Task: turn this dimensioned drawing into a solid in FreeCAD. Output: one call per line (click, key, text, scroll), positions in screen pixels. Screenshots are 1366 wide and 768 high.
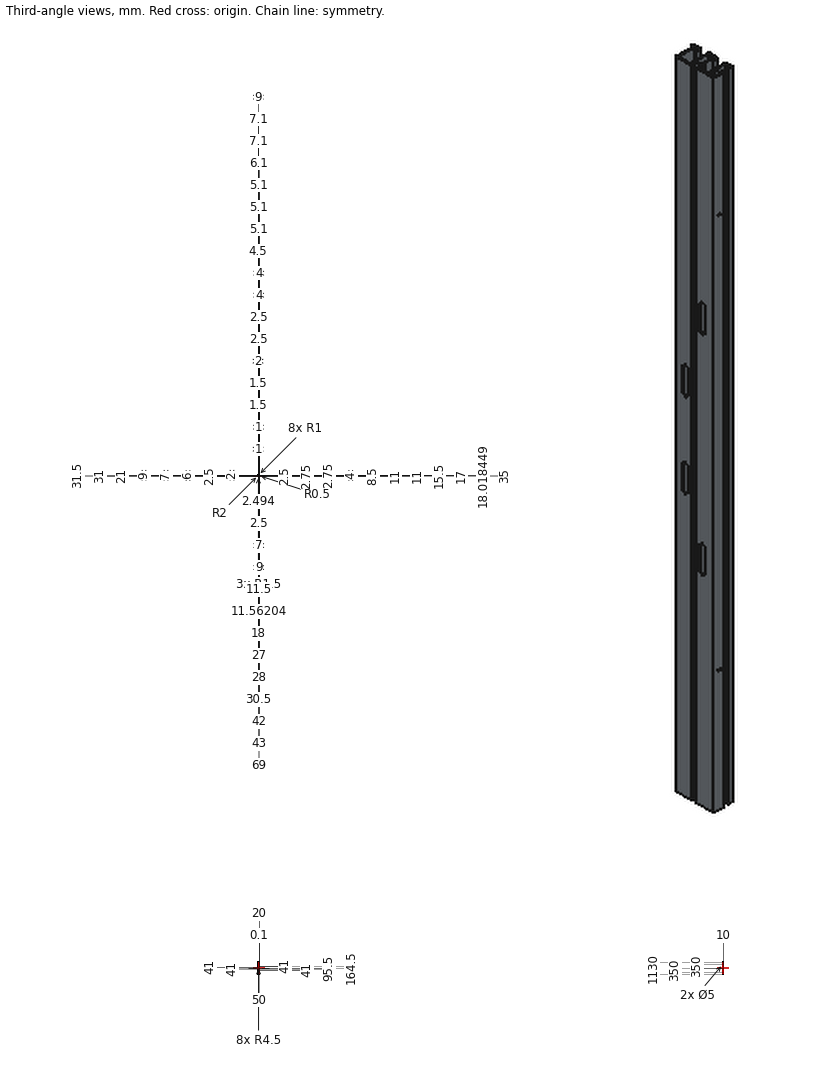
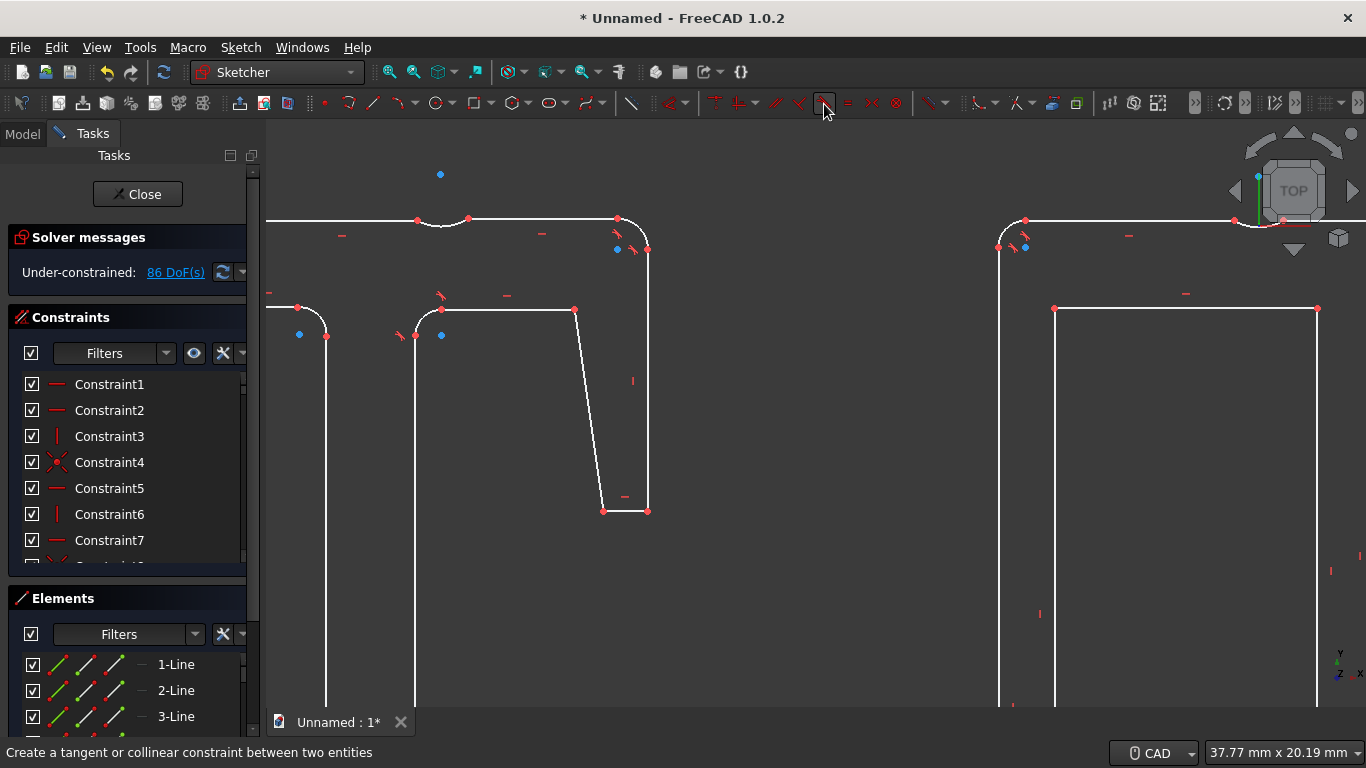
click(373, 221)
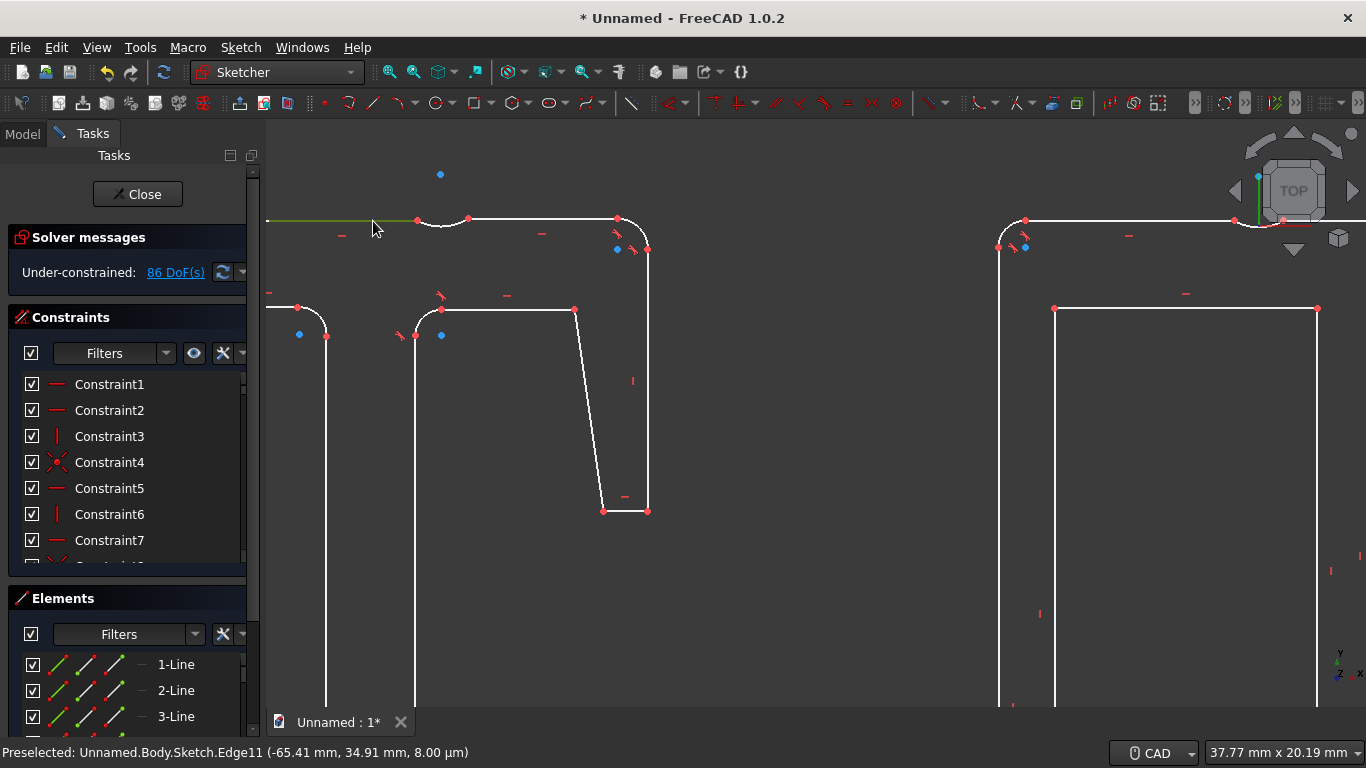
scroll(527, 277, down, 6)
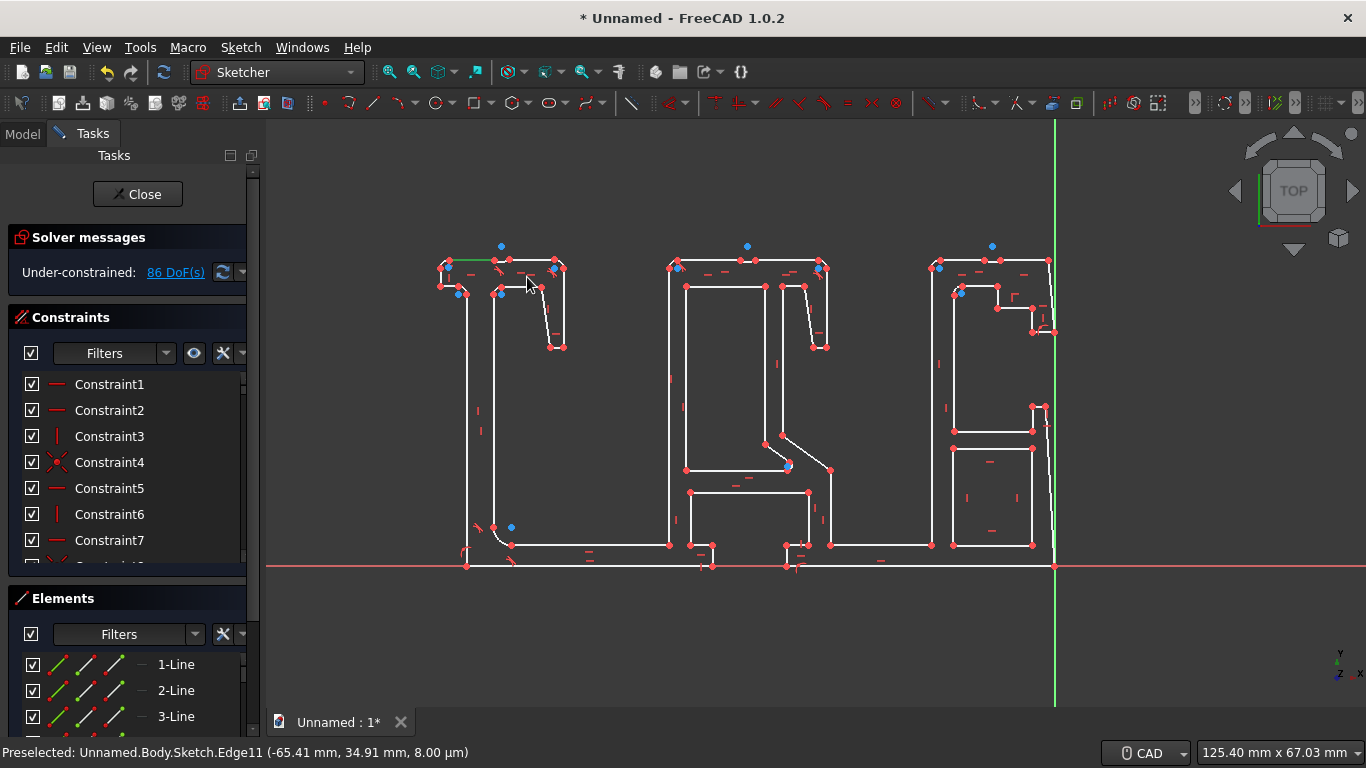
scroll(445, 261, up, 6)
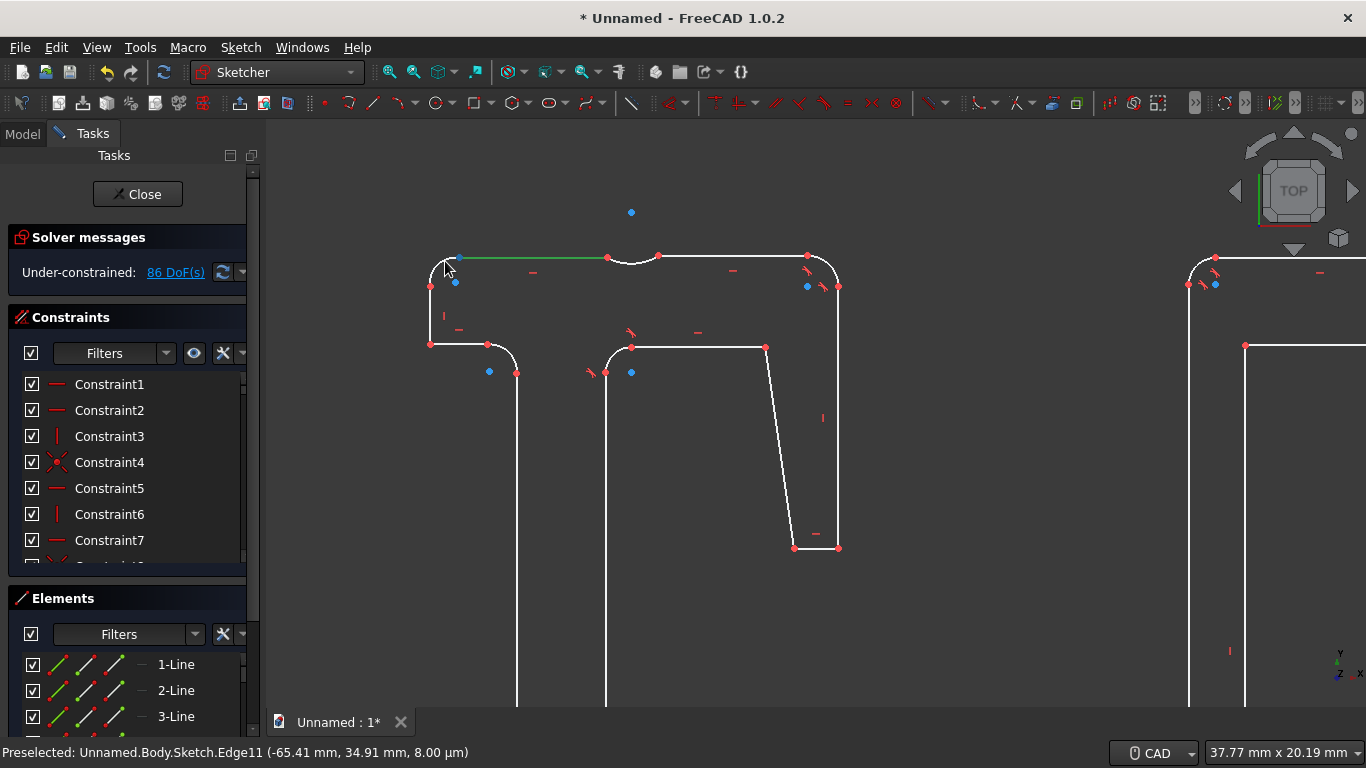
click(445, 260)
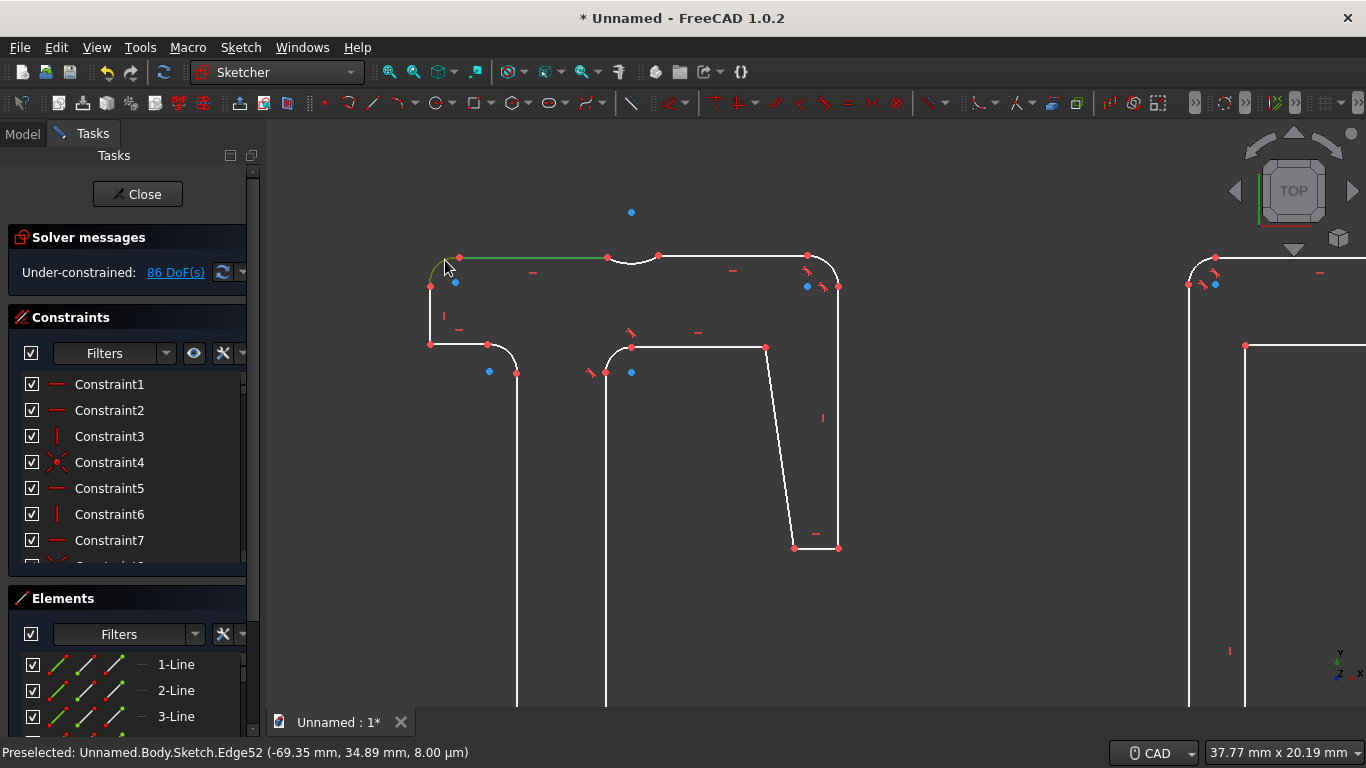
key(t)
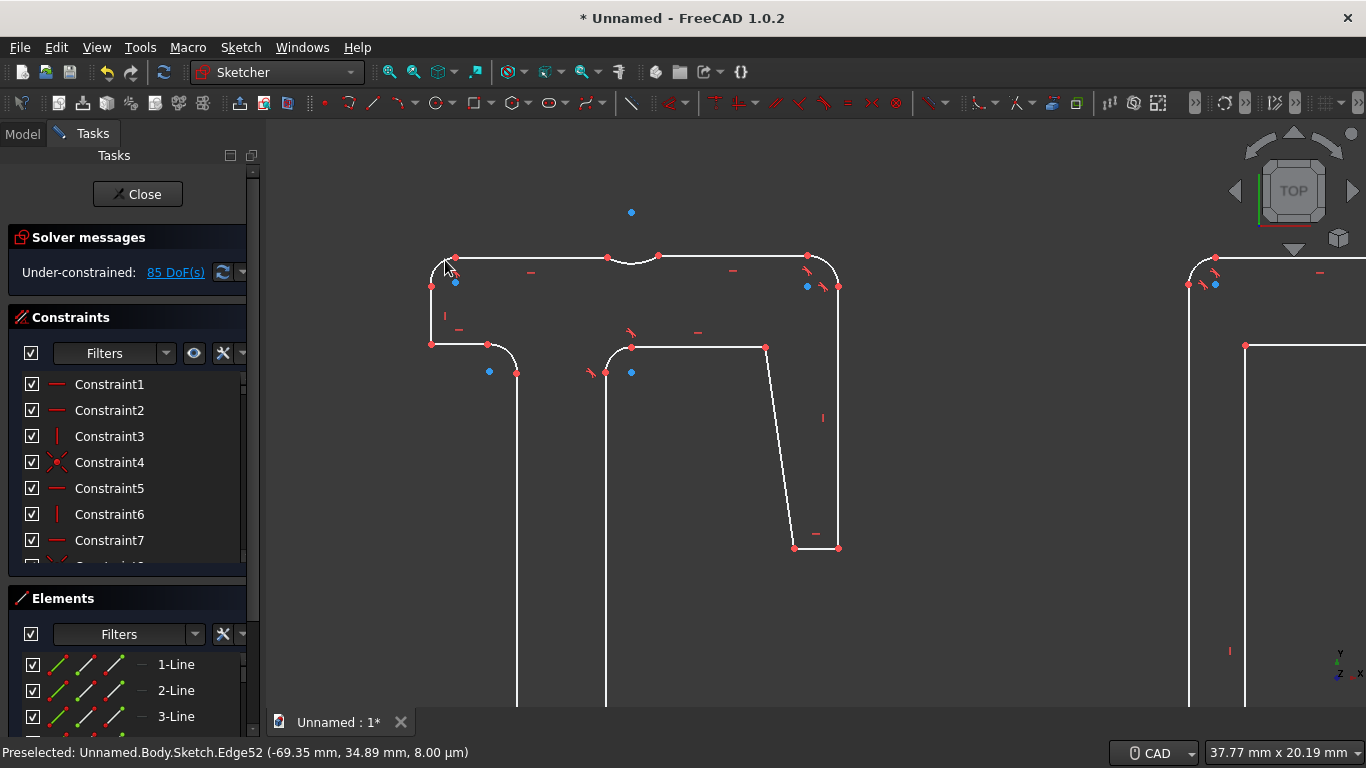
click(431, 304)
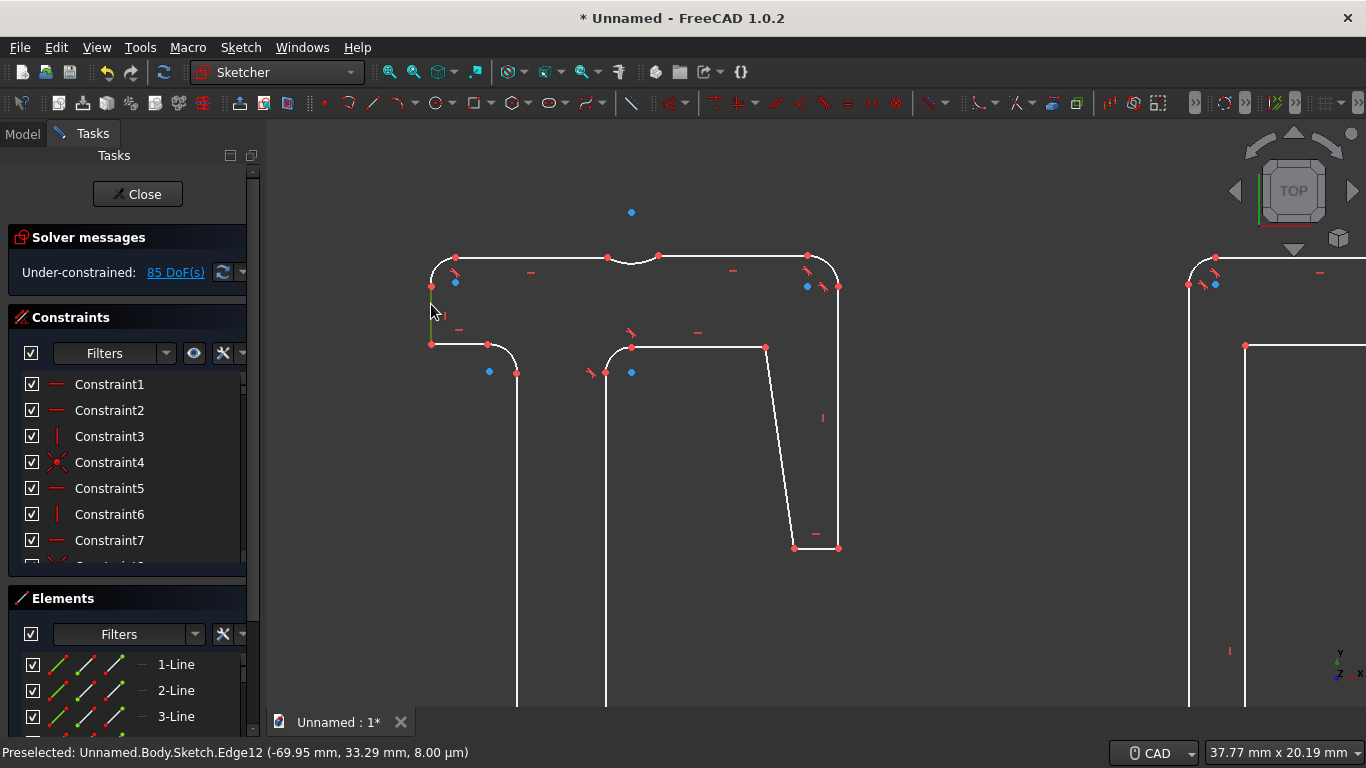
click(443, 261)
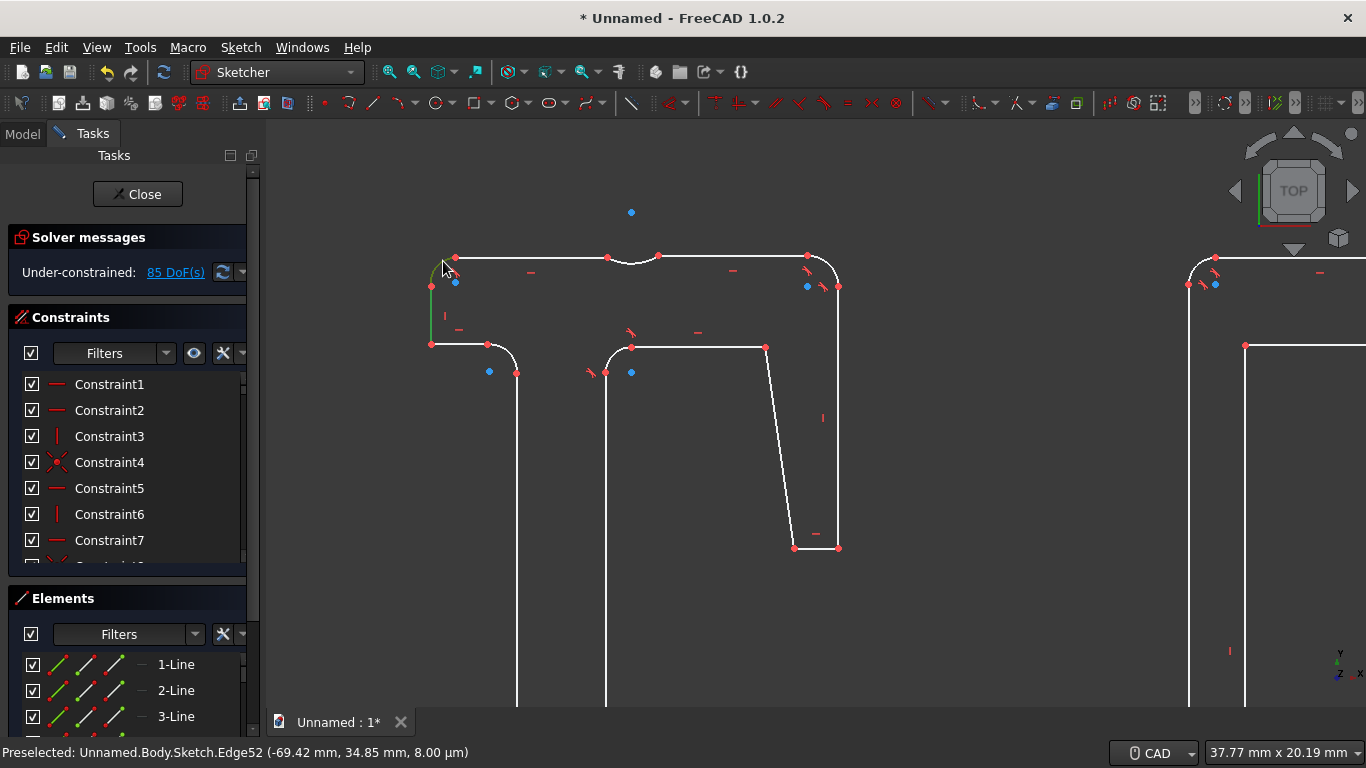
click(824, 104)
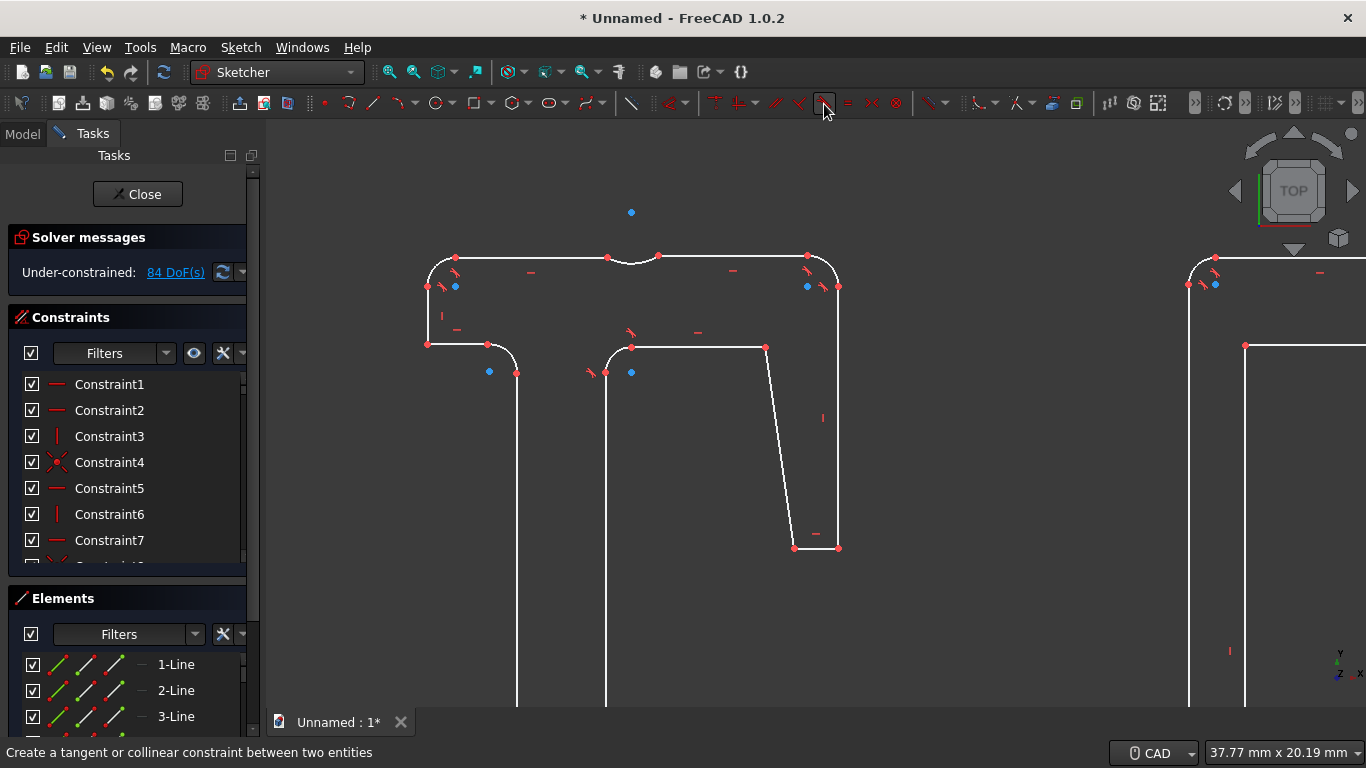
click(446, 344)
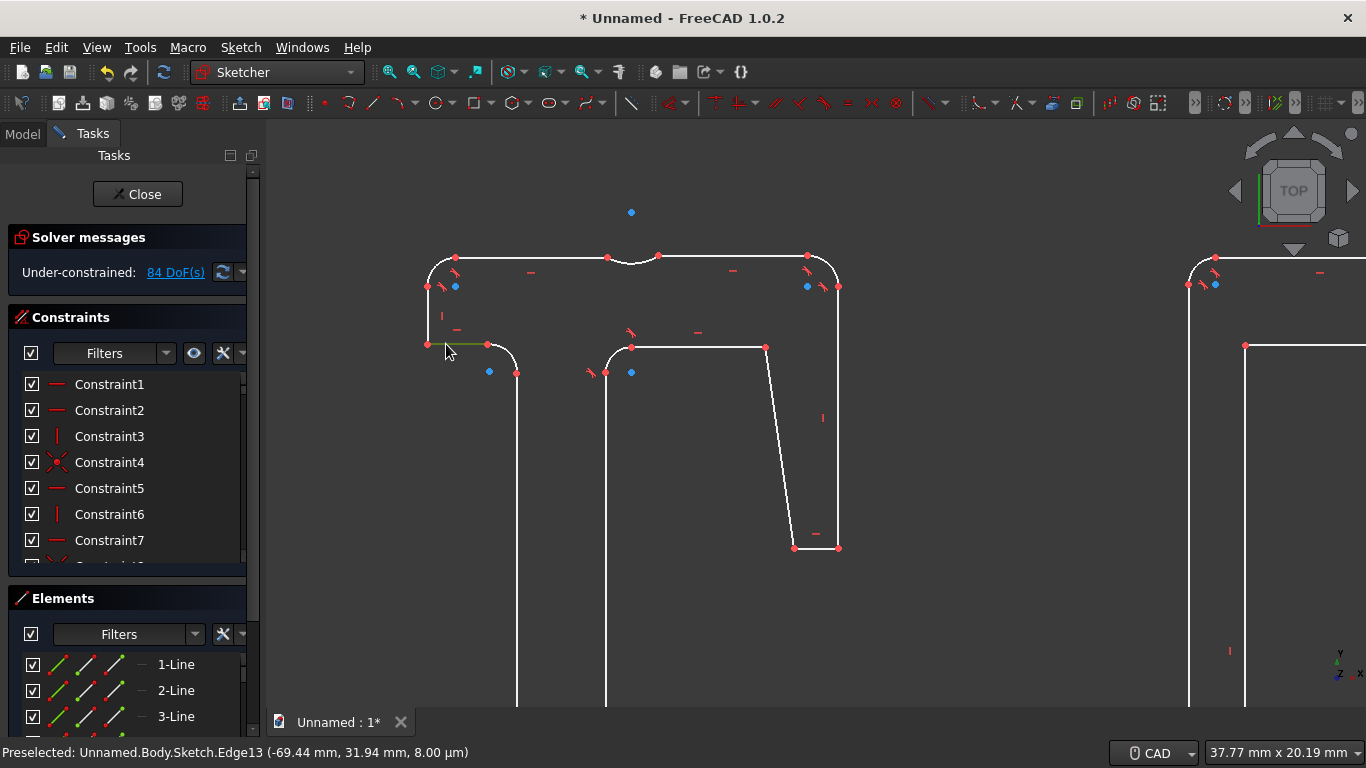
click(514, 360)